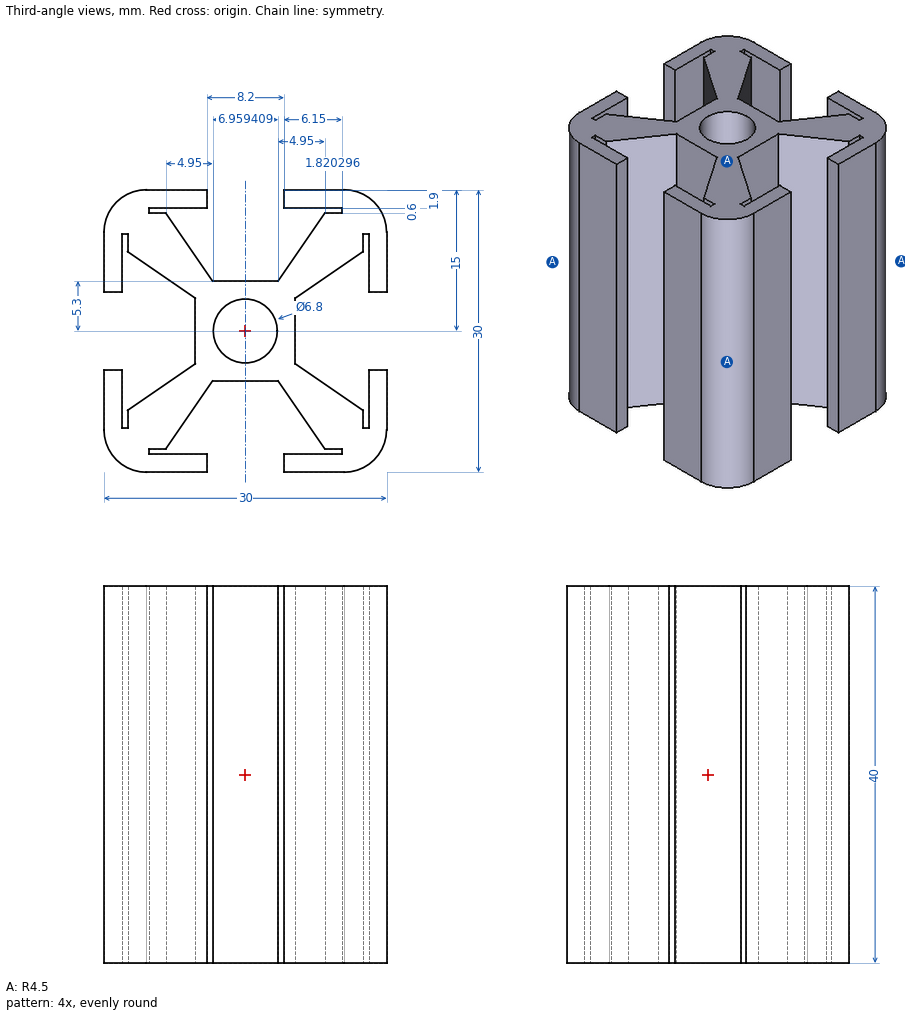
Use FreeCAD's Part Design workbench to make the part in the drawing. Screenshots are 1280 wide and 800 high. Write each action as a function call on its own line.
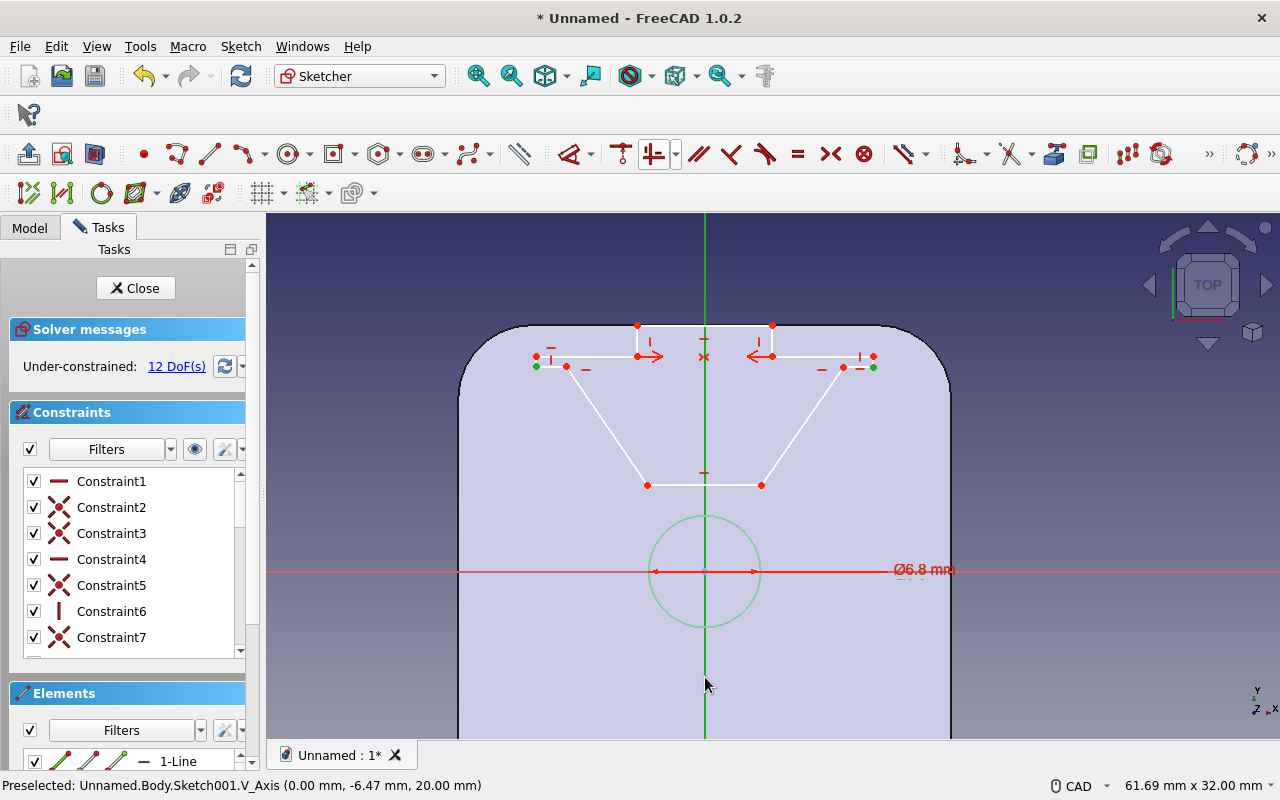
key(s)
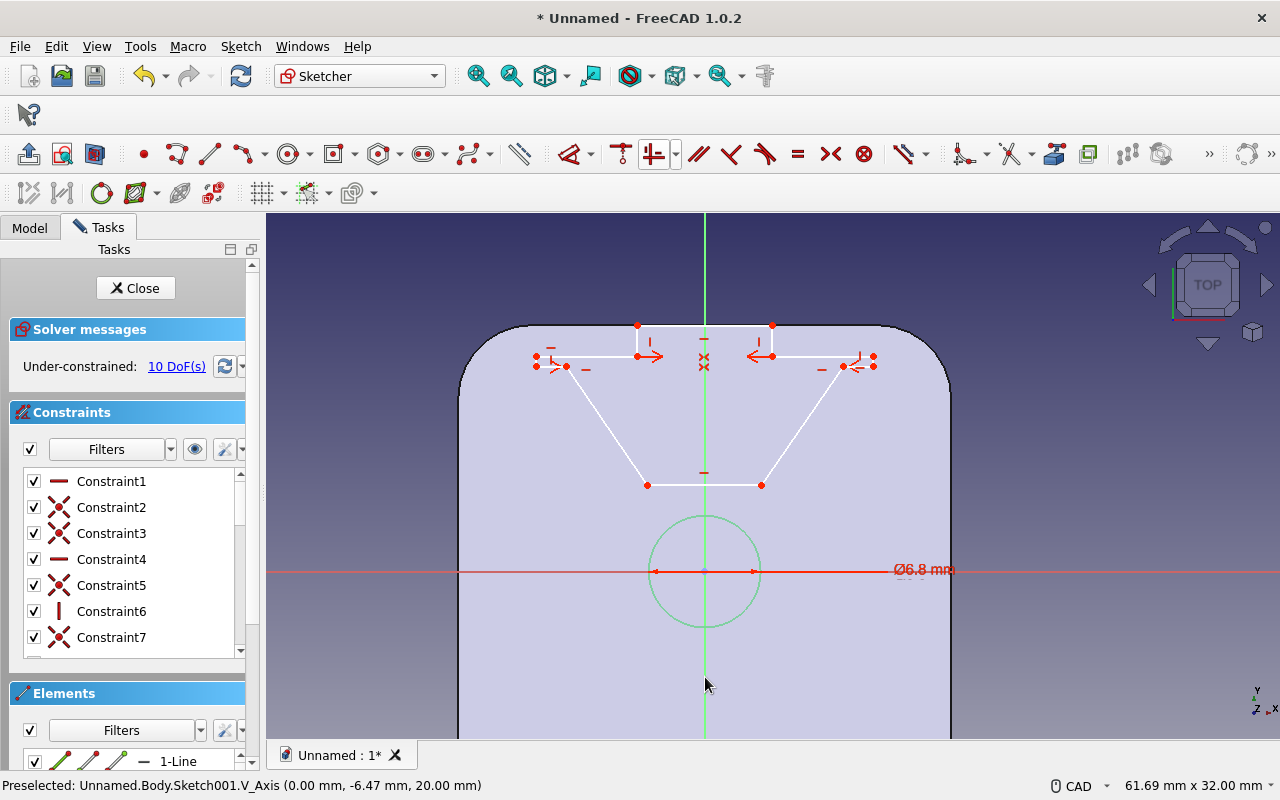
key(d)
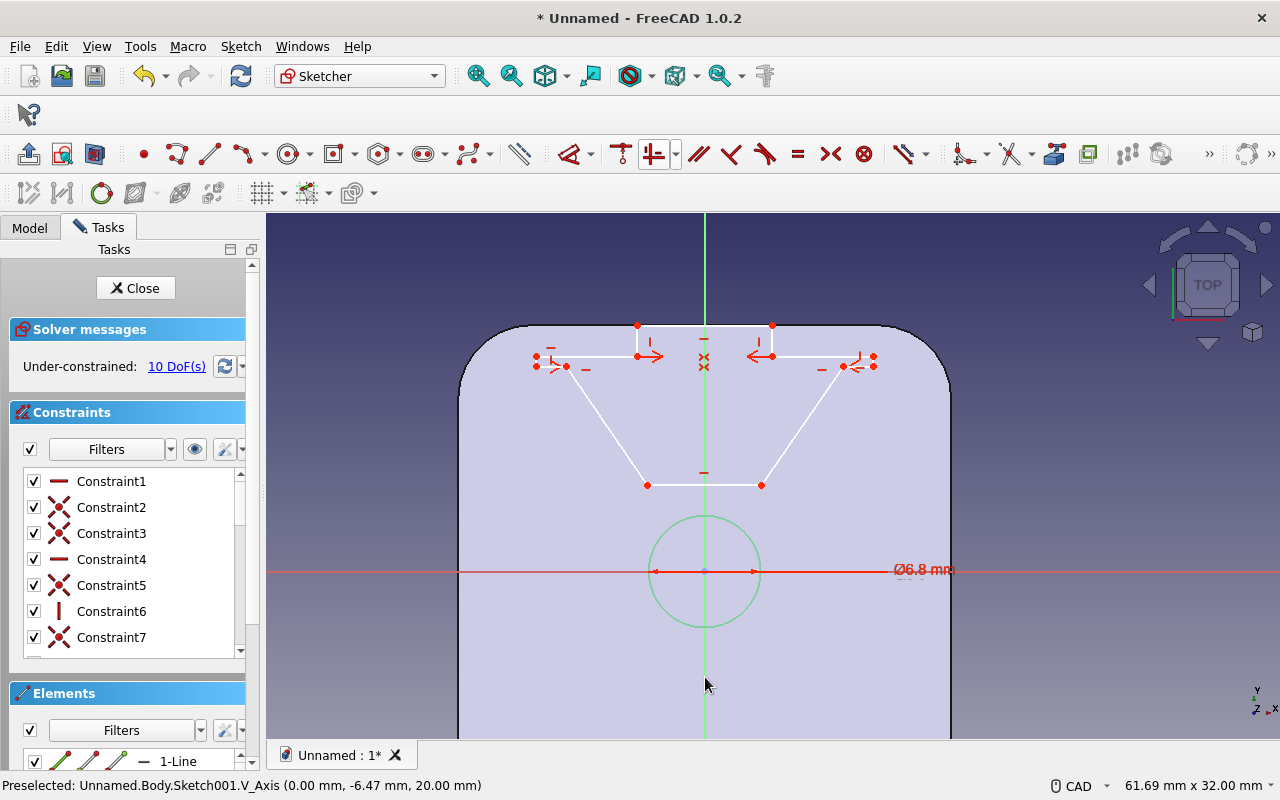
scroll(873, 362, up, 7)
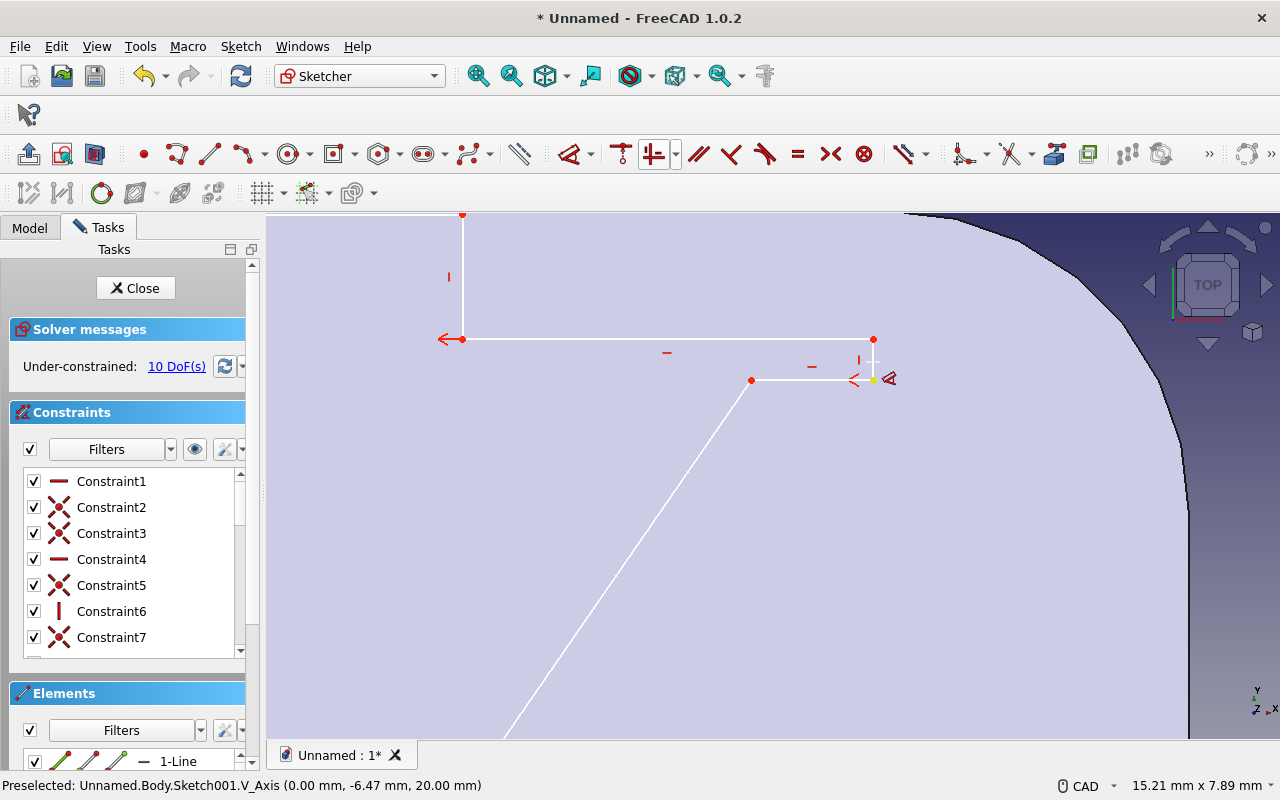
click(873, 360)
click(907, 360)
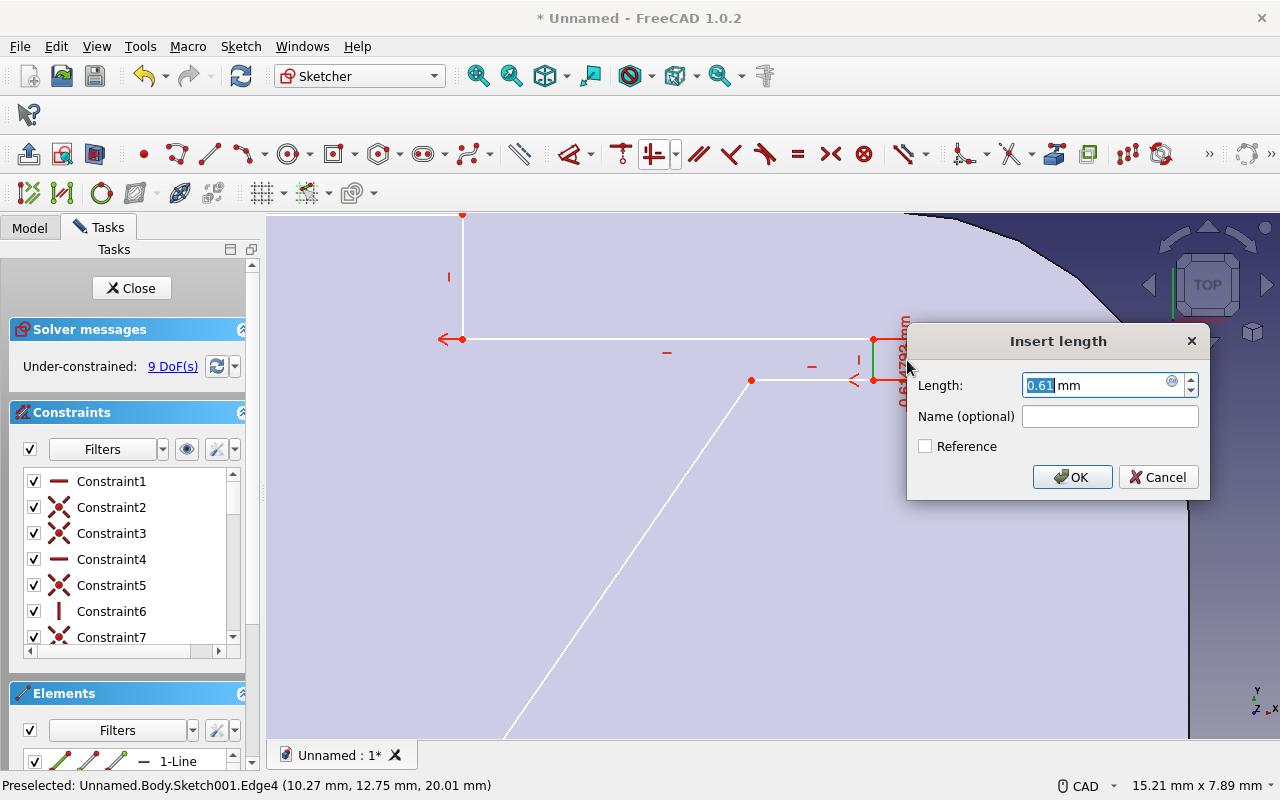
text(0.6)
key(Return)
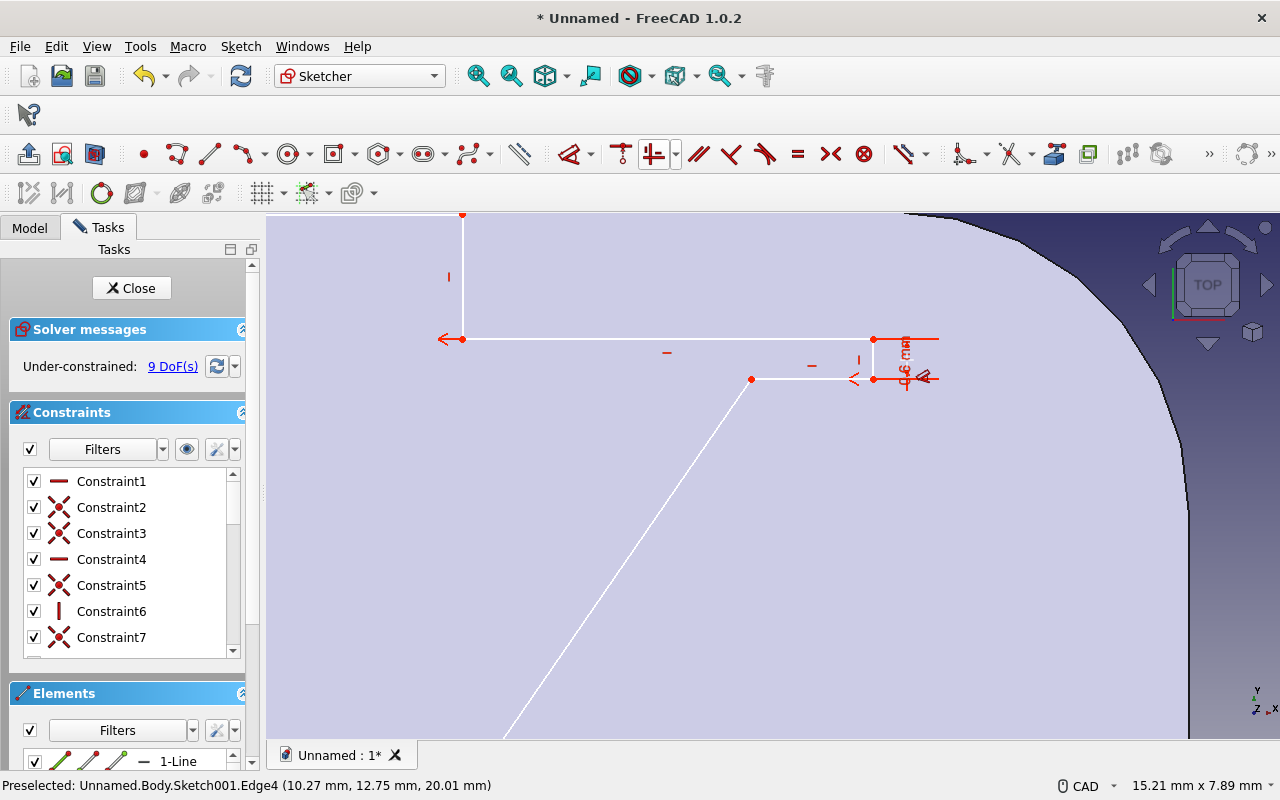
click(463, 302)
click(497, 290)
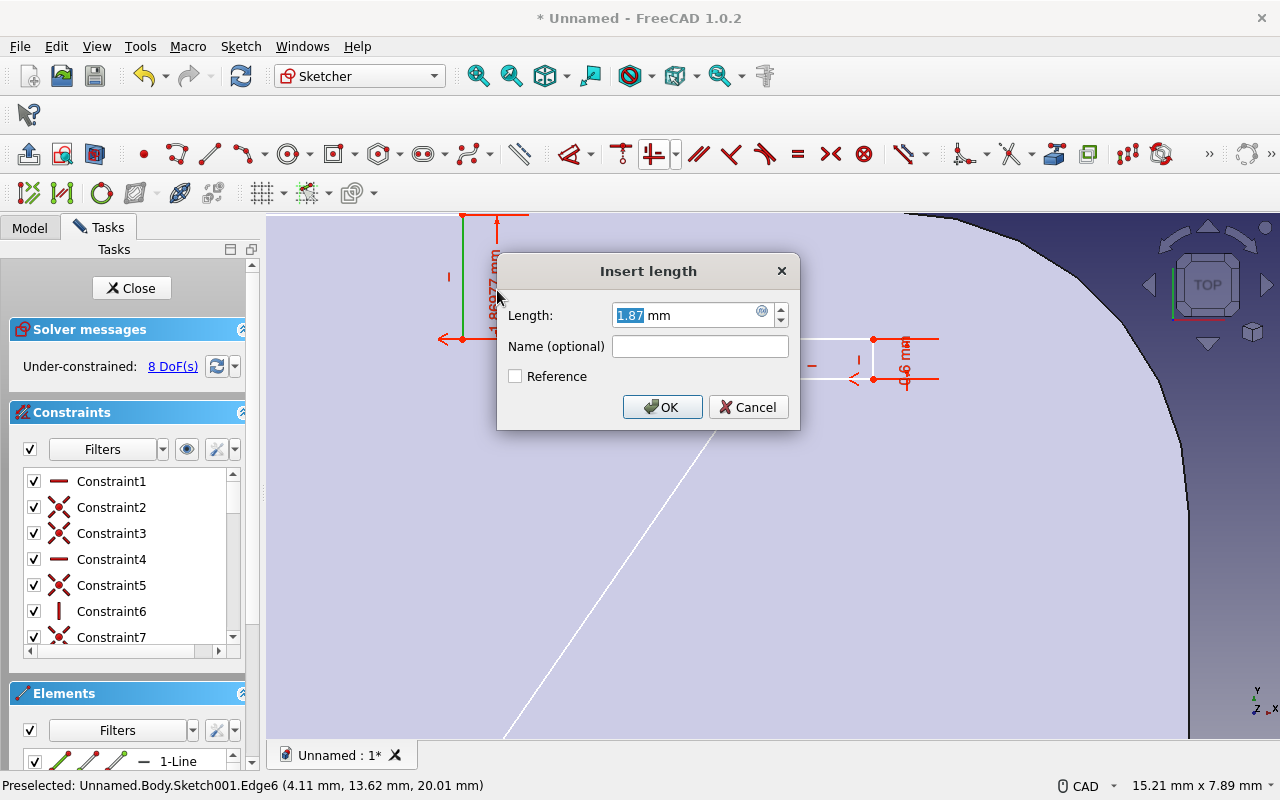
text(1.9)
key(Return)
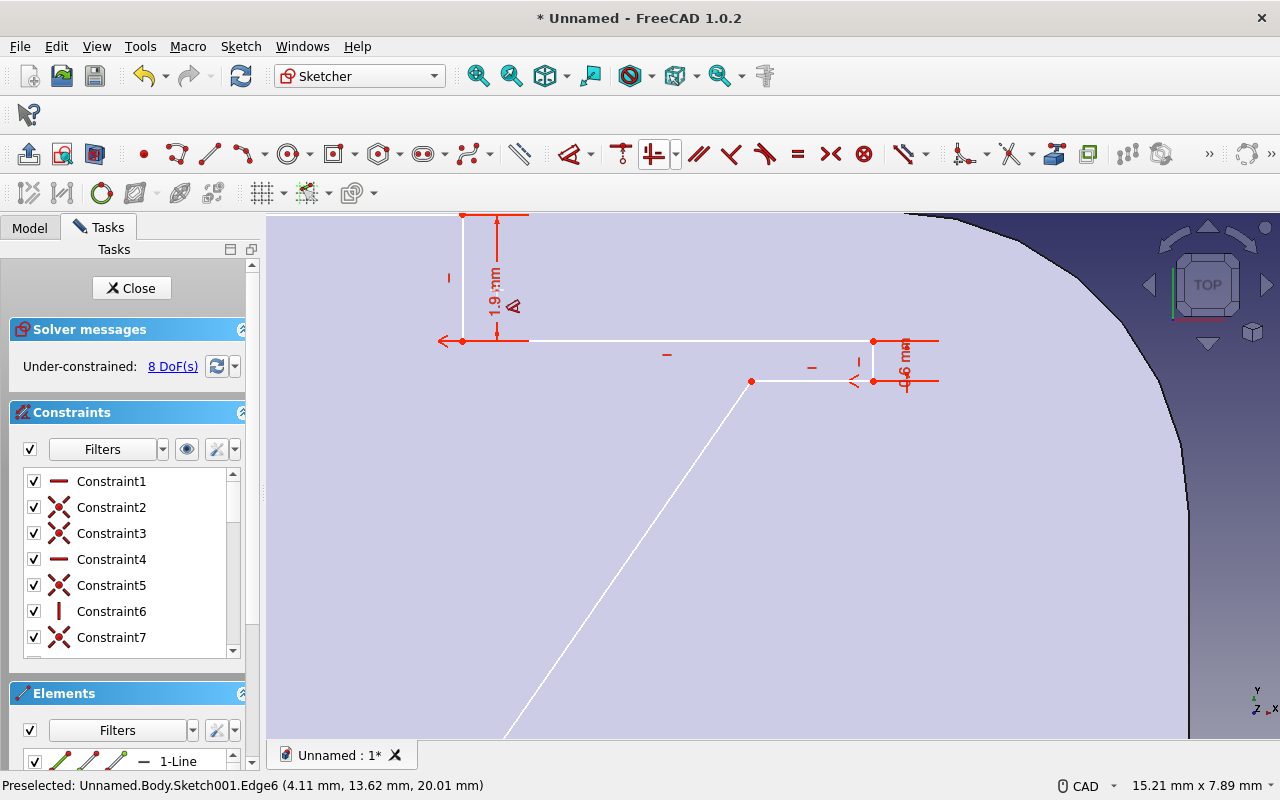
scroll(873, 362, down, 7)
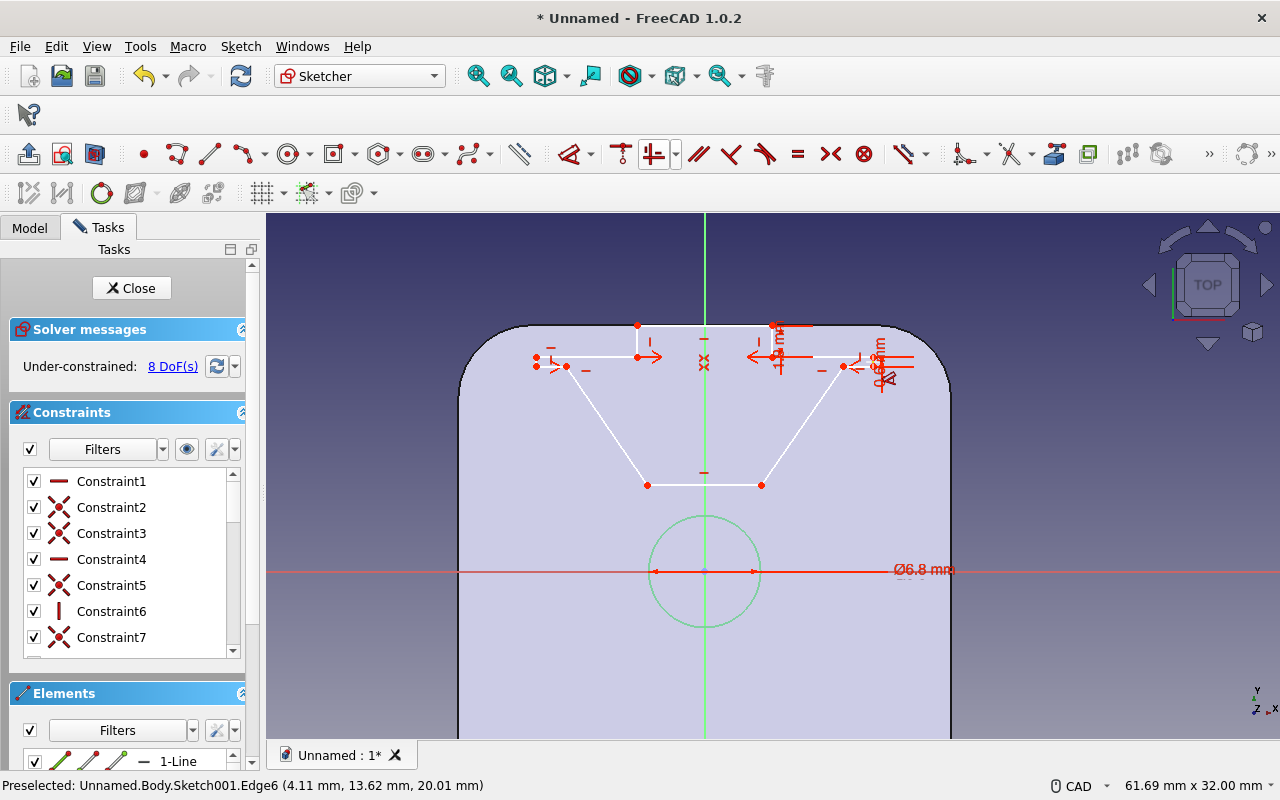
click(732, 326)
click(674, 292)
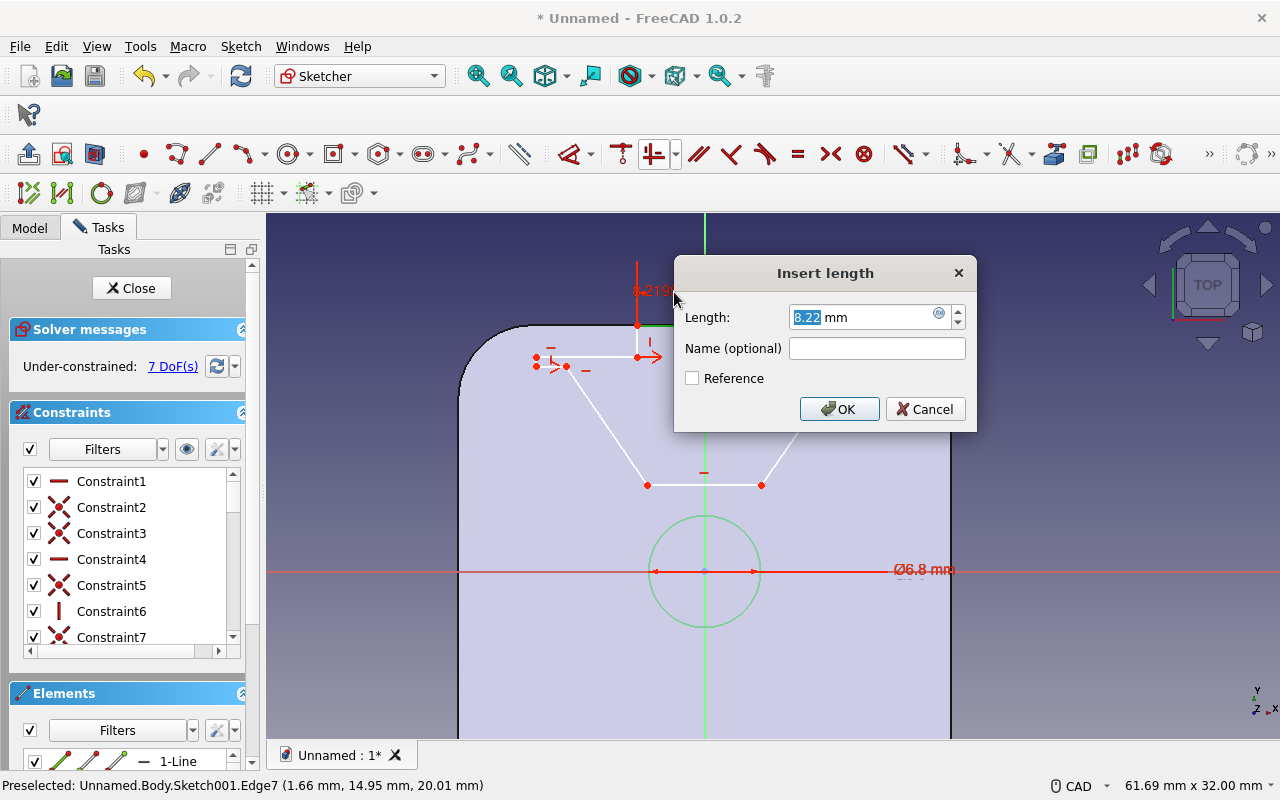
text(8.2)
key(Return)